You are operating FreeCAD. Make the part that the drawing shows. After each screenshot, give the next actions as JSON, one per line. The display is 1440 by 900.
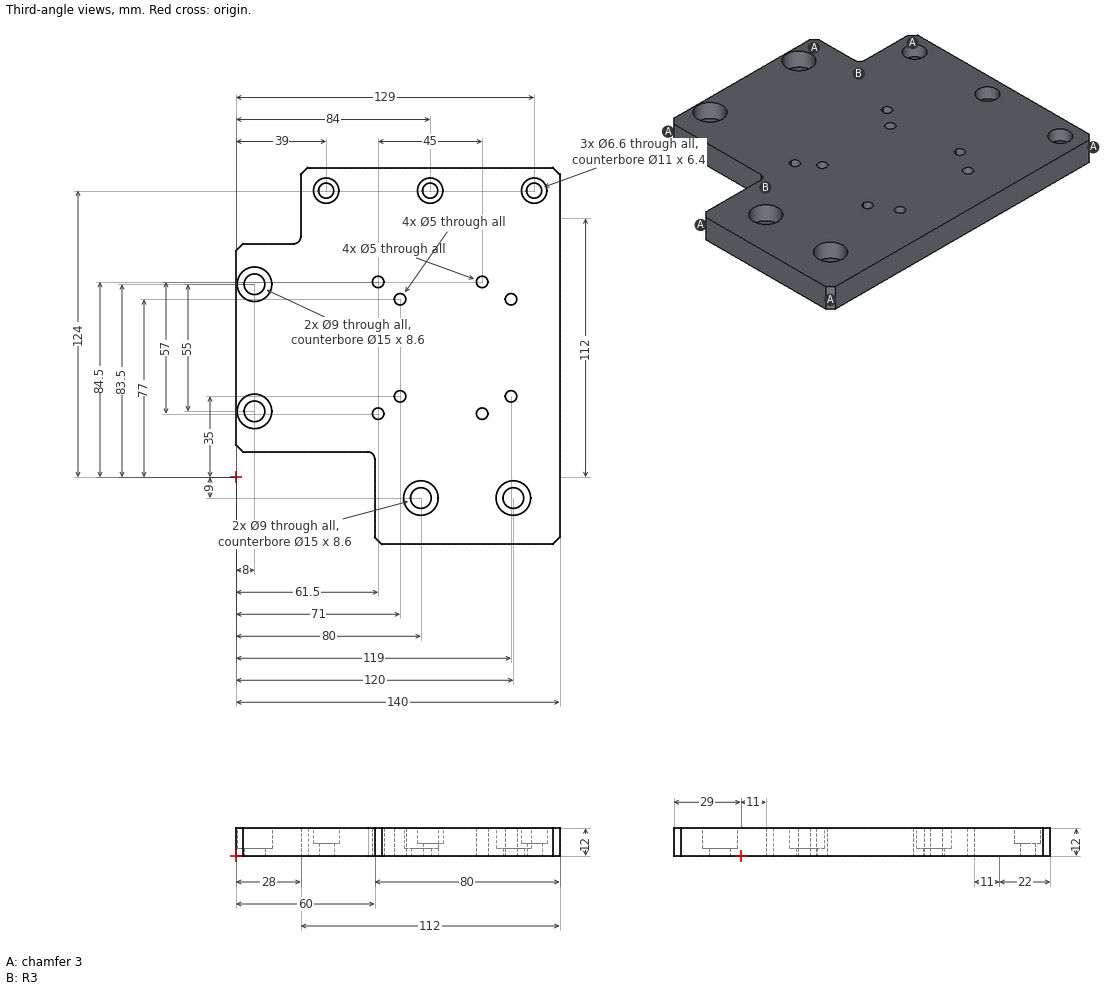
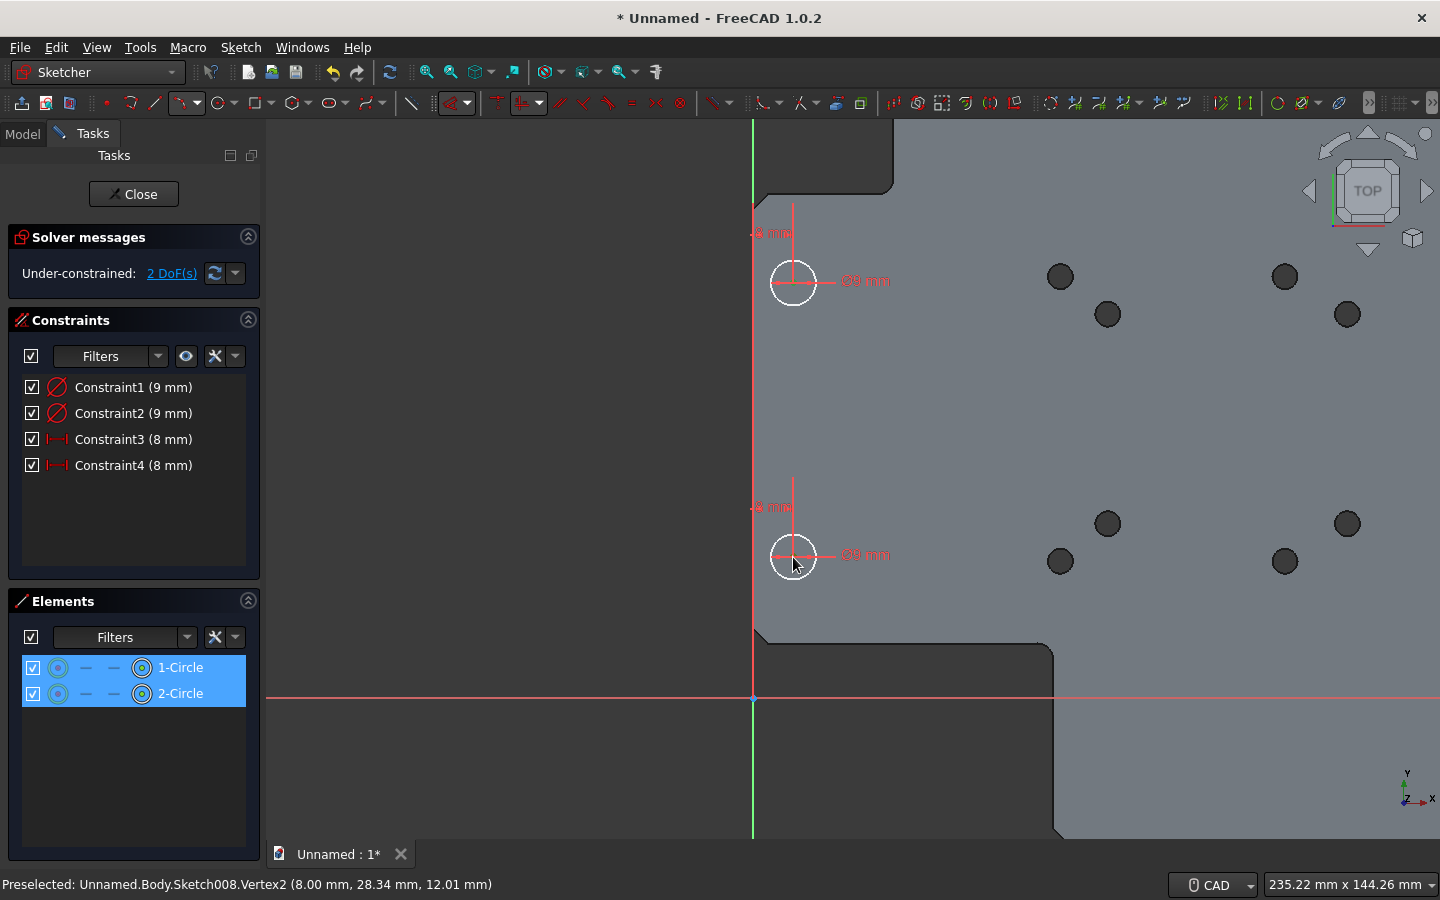
{"action": "key", "text": "i"}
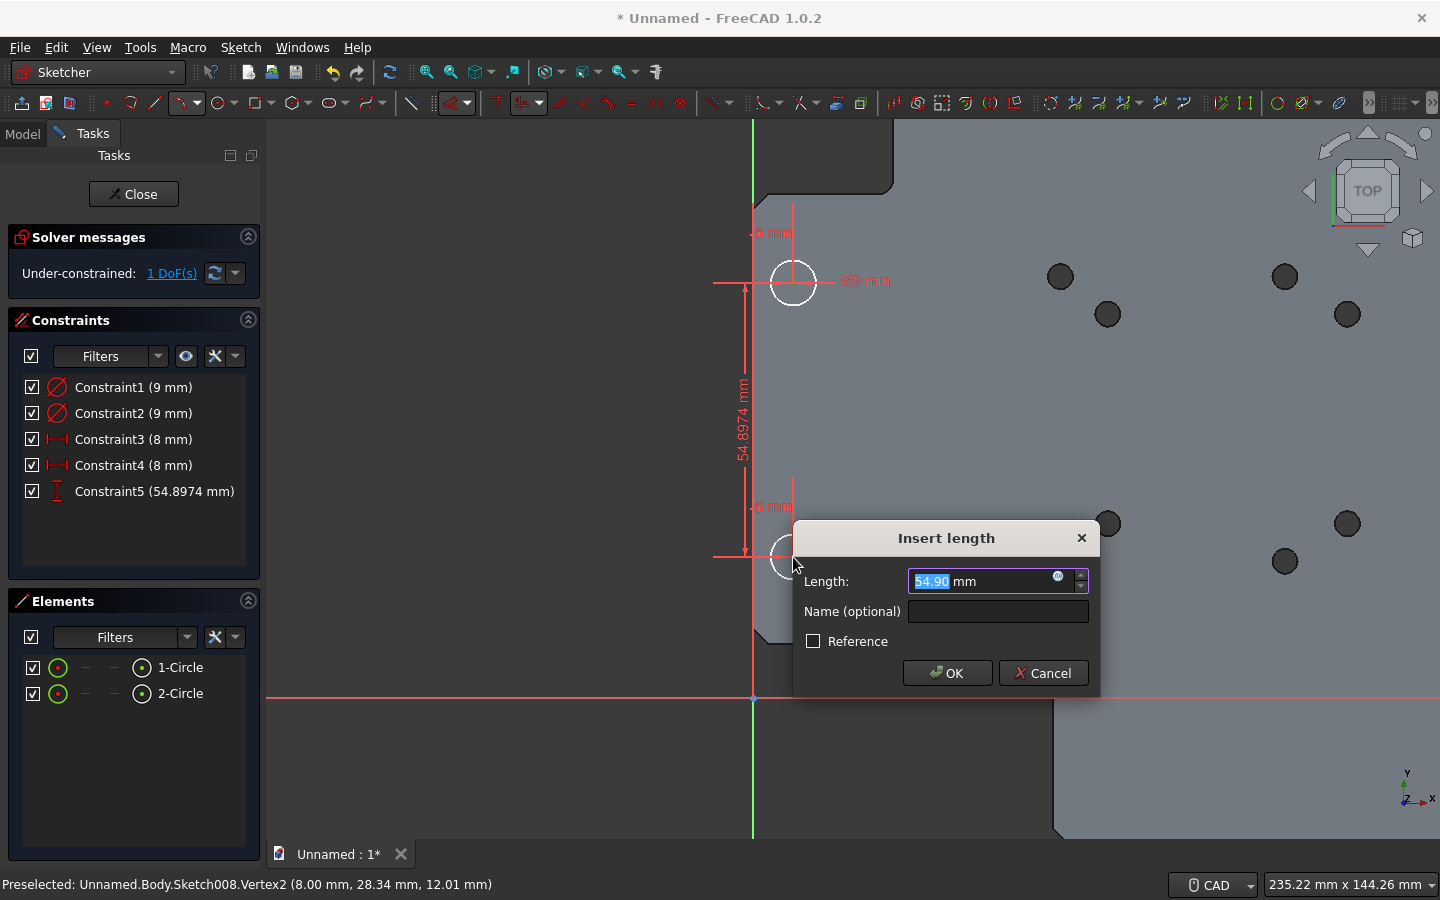
{"action": "type", "text": "55"}
{"action": "key", "text": "Return"}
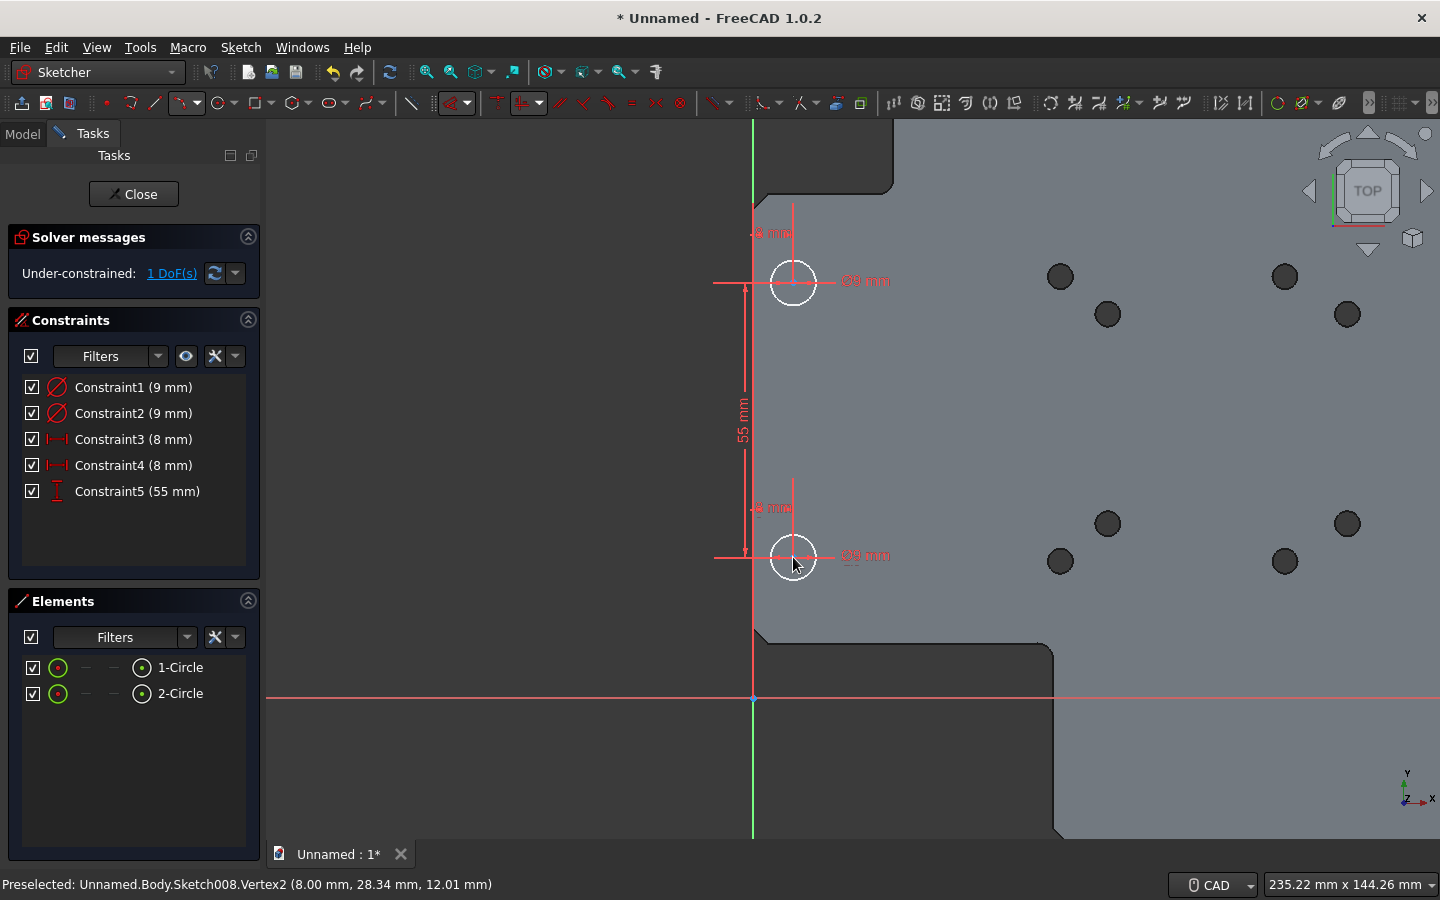
{"action": "left_click", "coordinate": [793, 283]}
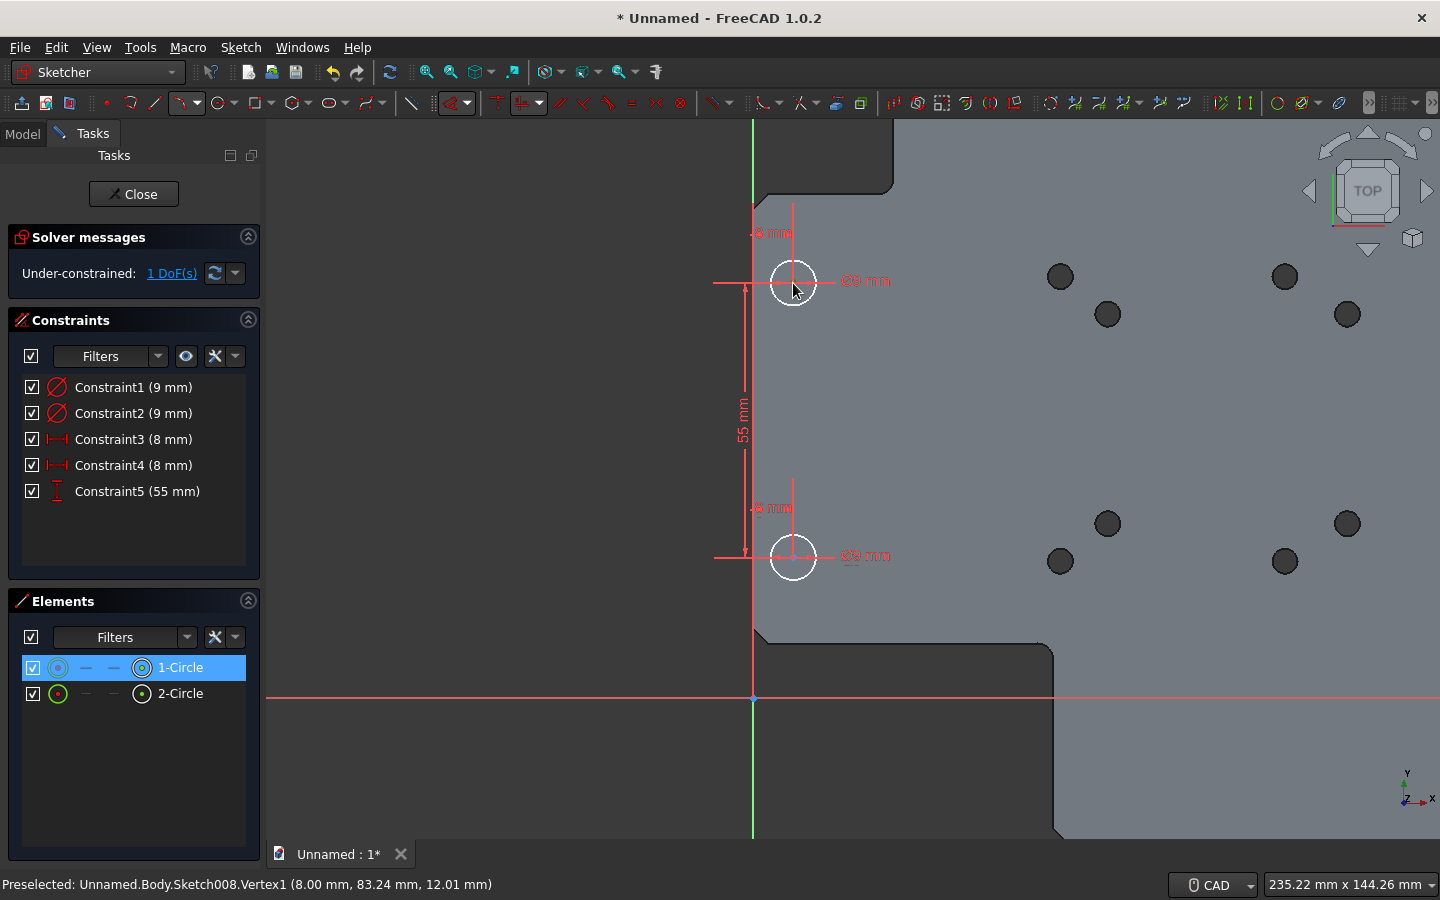
{"action": "left_click", "coordinate": [470, 104]}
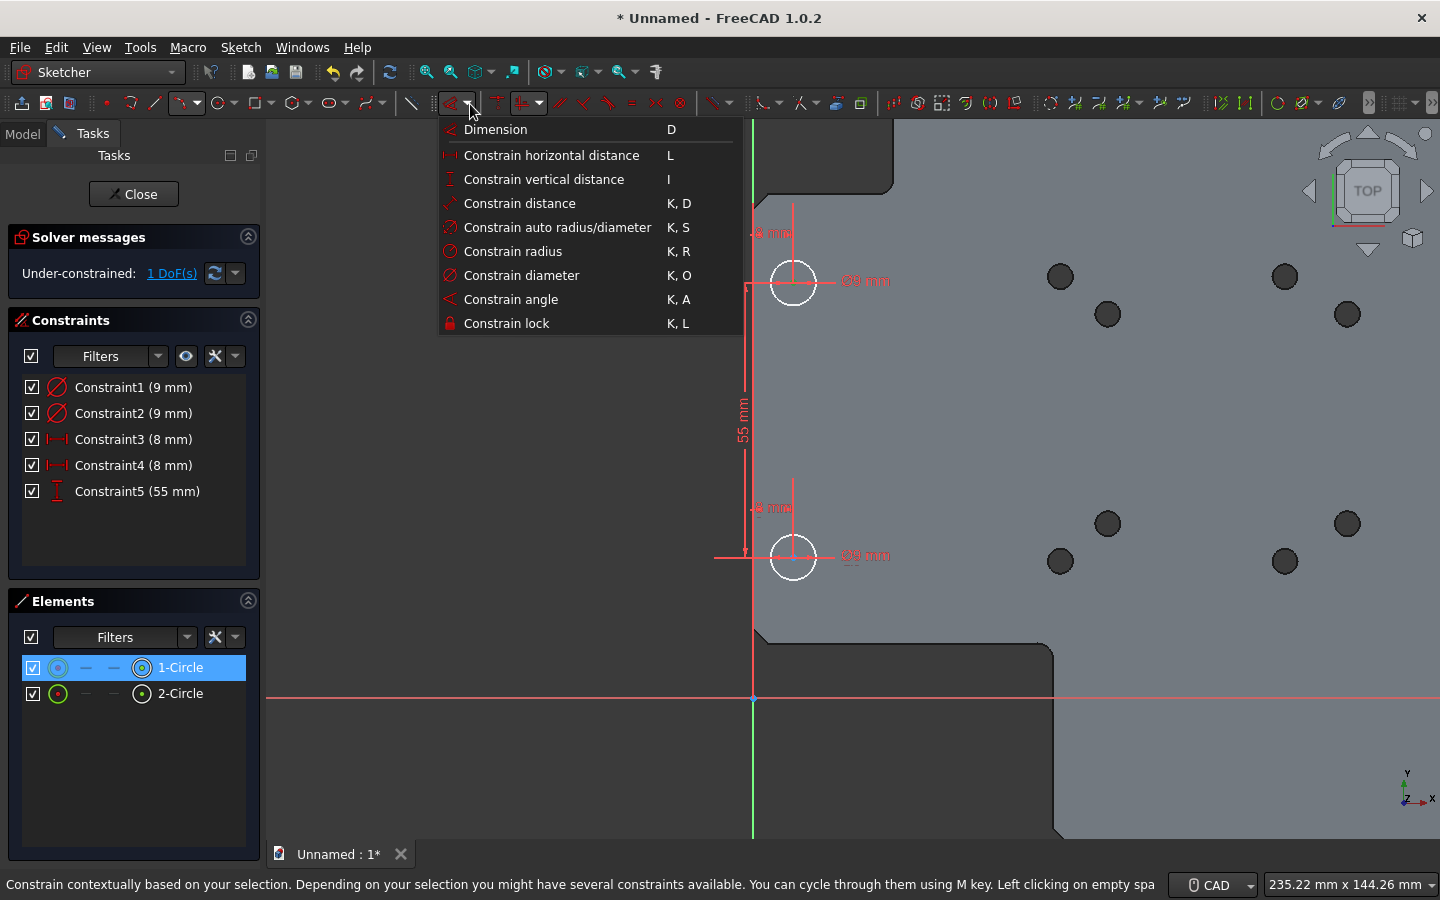
{"action": "left_click", "coordinate": [591, 179]}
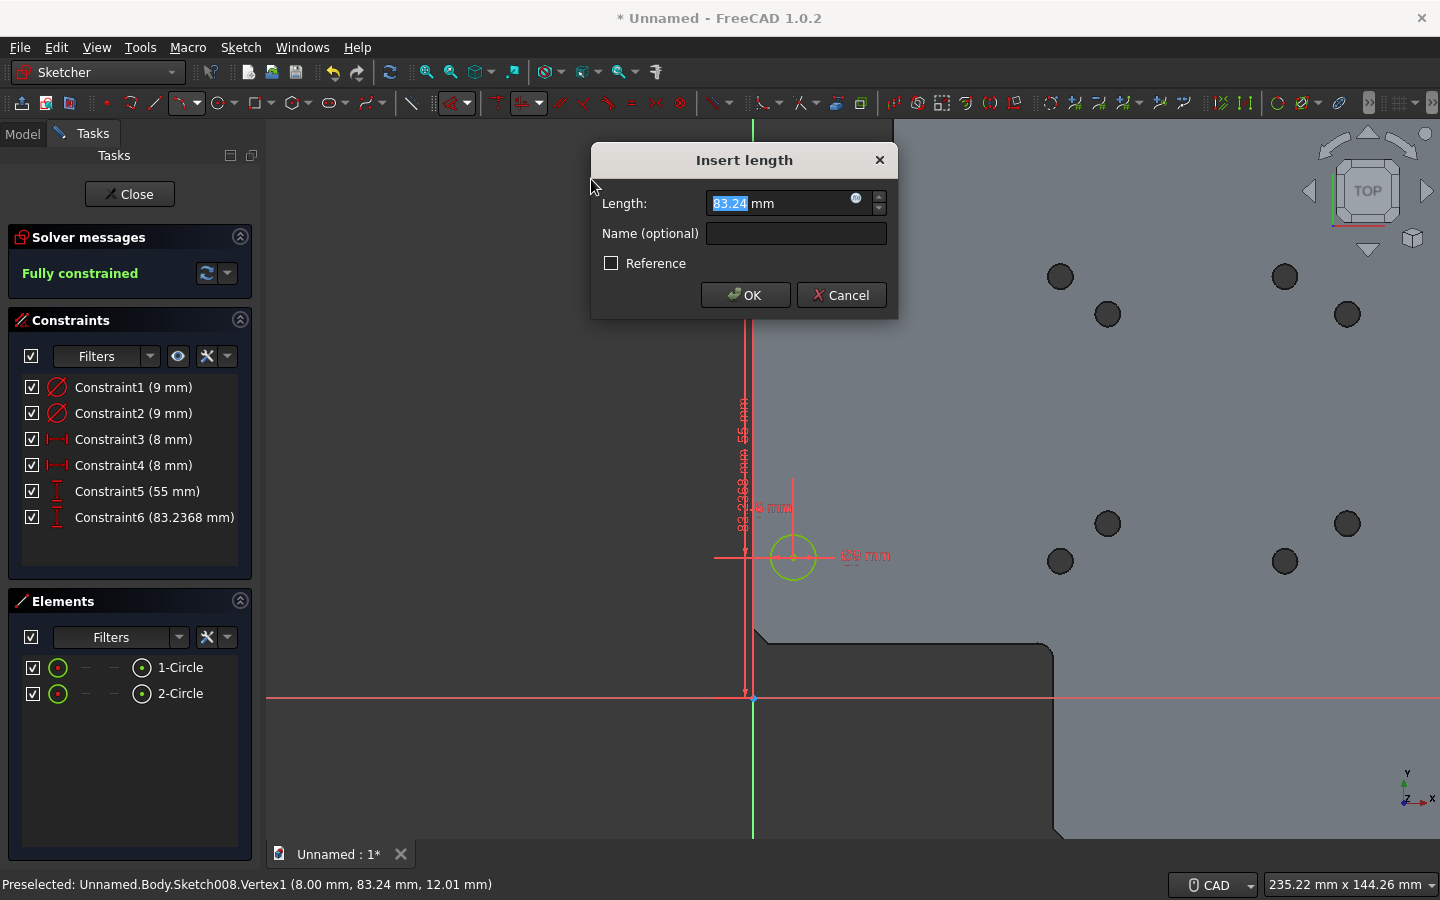
{"action": "type", "text": "83.5"}
{"action": "key", "text": "Return"}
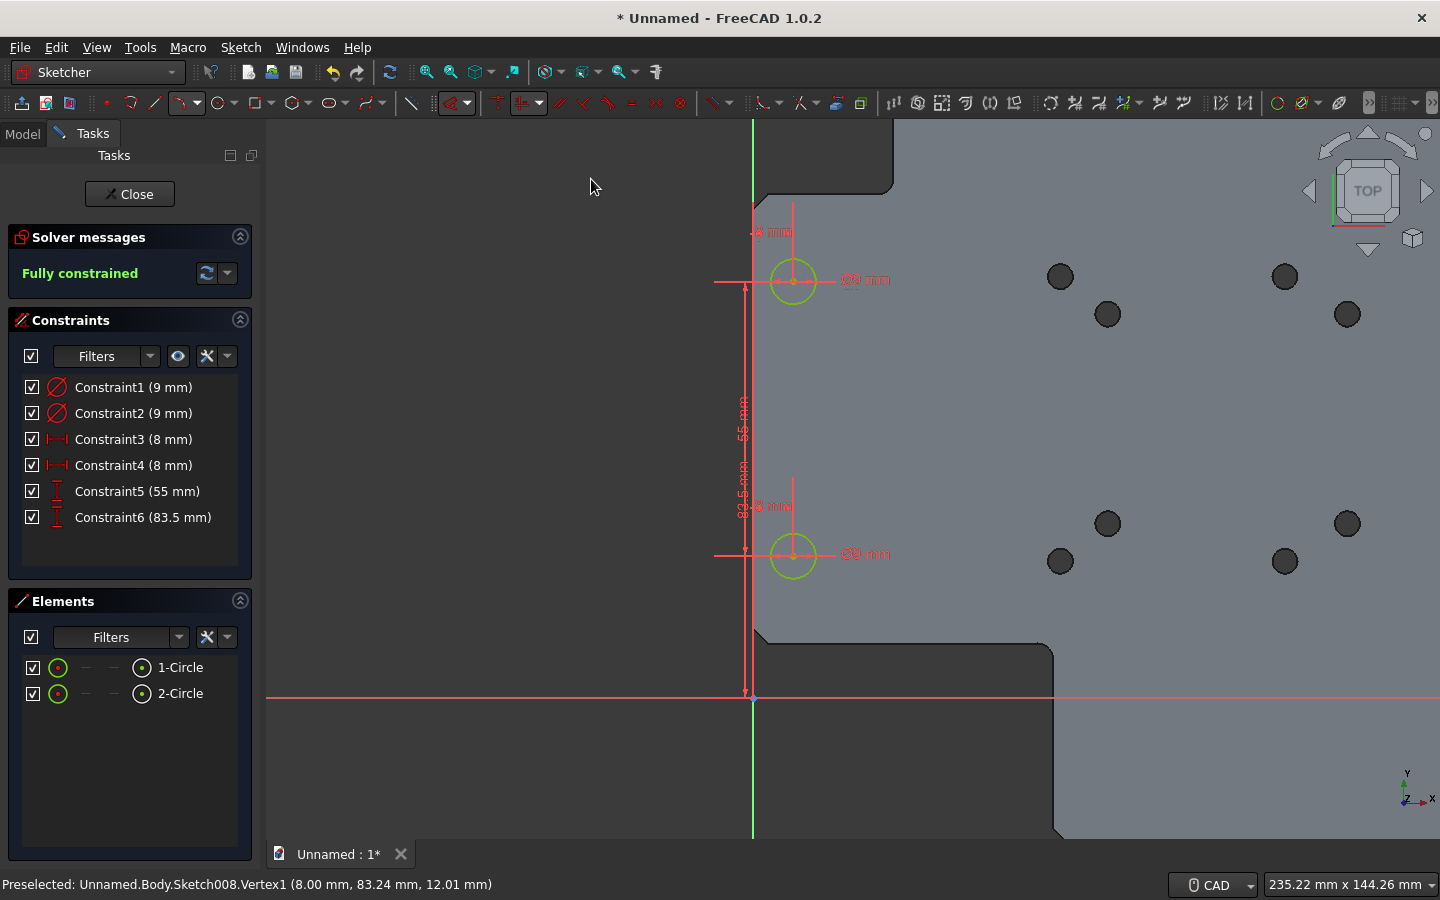
{"action": "left_click", "coordinate": [130, 194]}